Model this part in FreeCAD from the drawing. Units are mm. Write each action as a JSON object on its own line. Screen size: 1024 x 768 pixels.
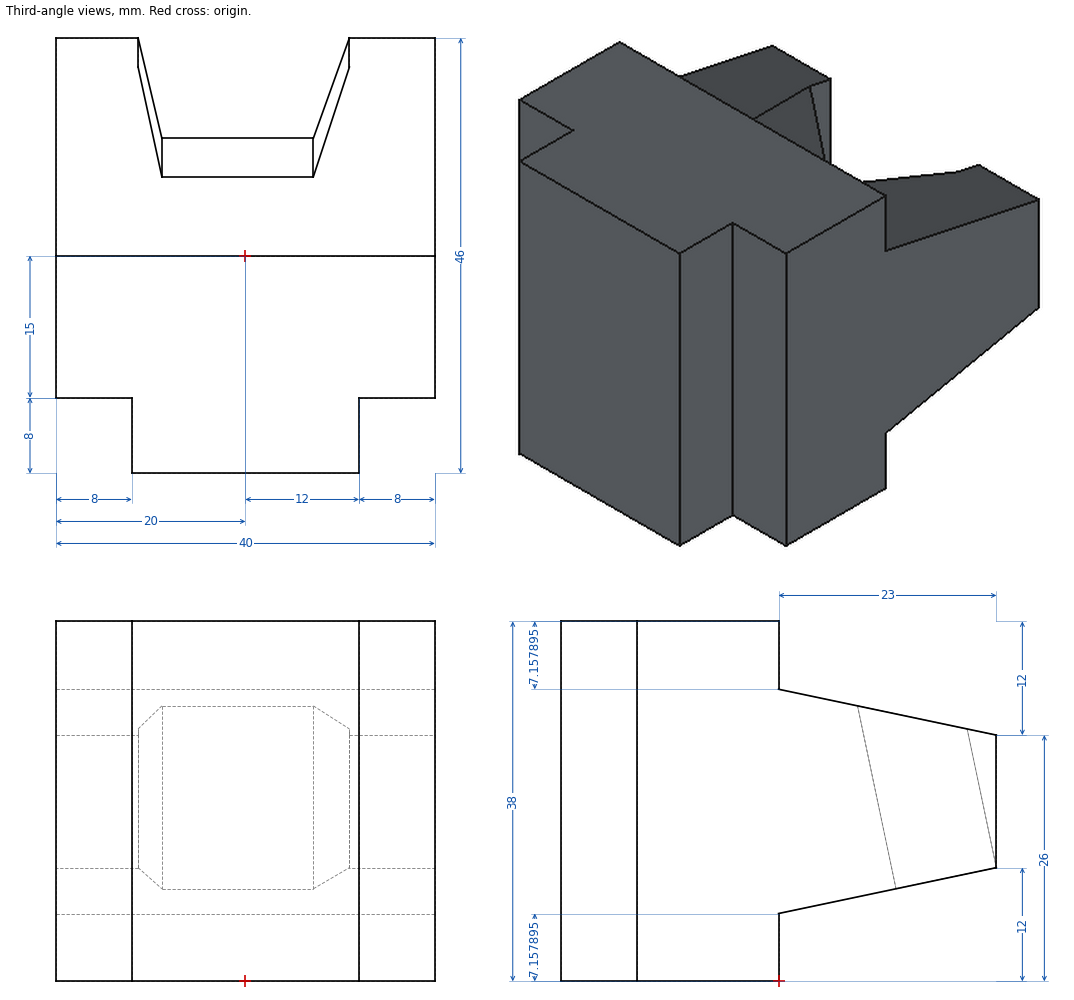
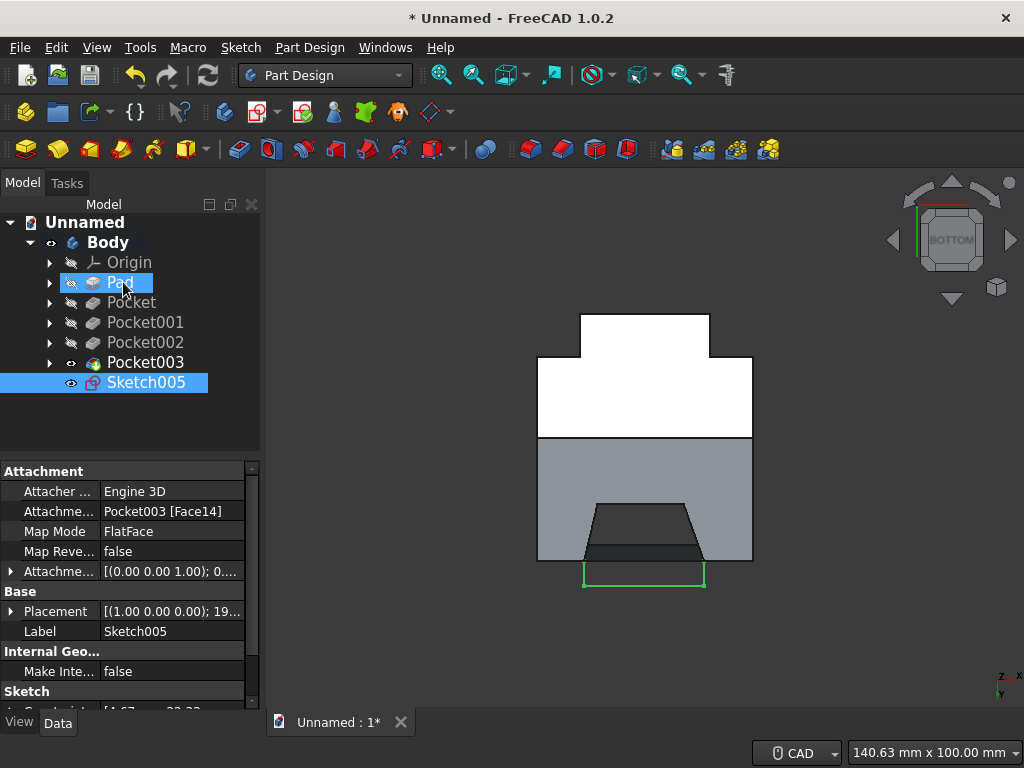
{"action": "left_click", "coordinate": [240, 150]}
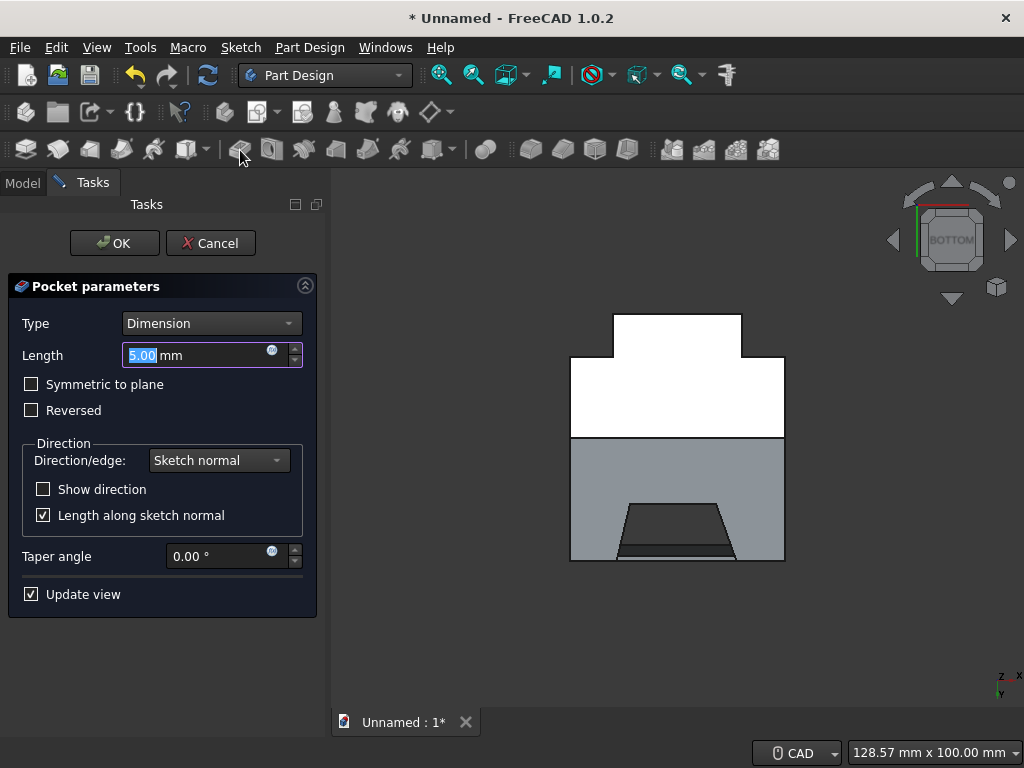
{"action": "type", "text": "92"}
{"action": "key", "text": "Tab"}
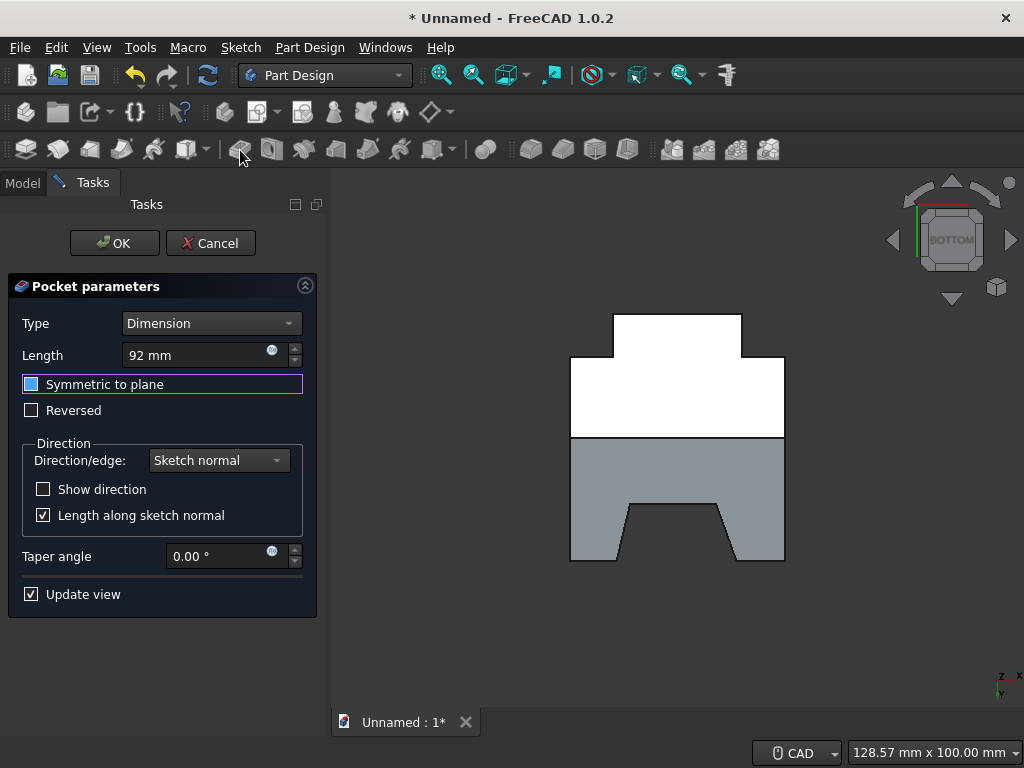
{"action": "left_click", "coordinate": [30, 384]}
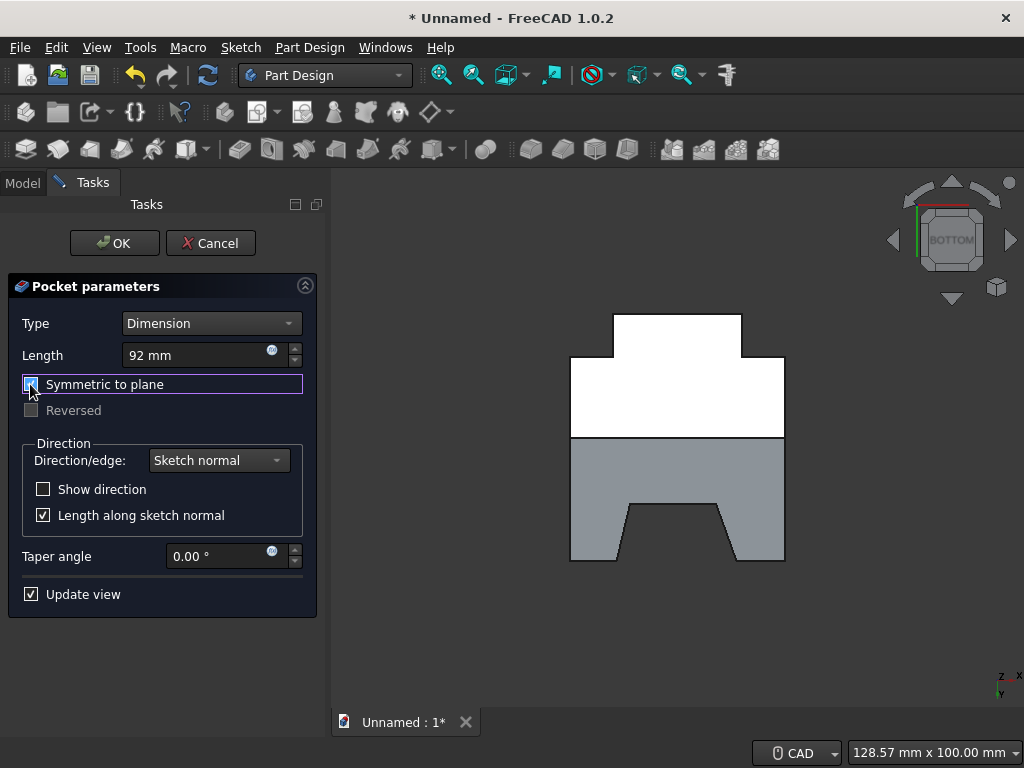
{"action": "left_click", "coordinate": [115, 243]}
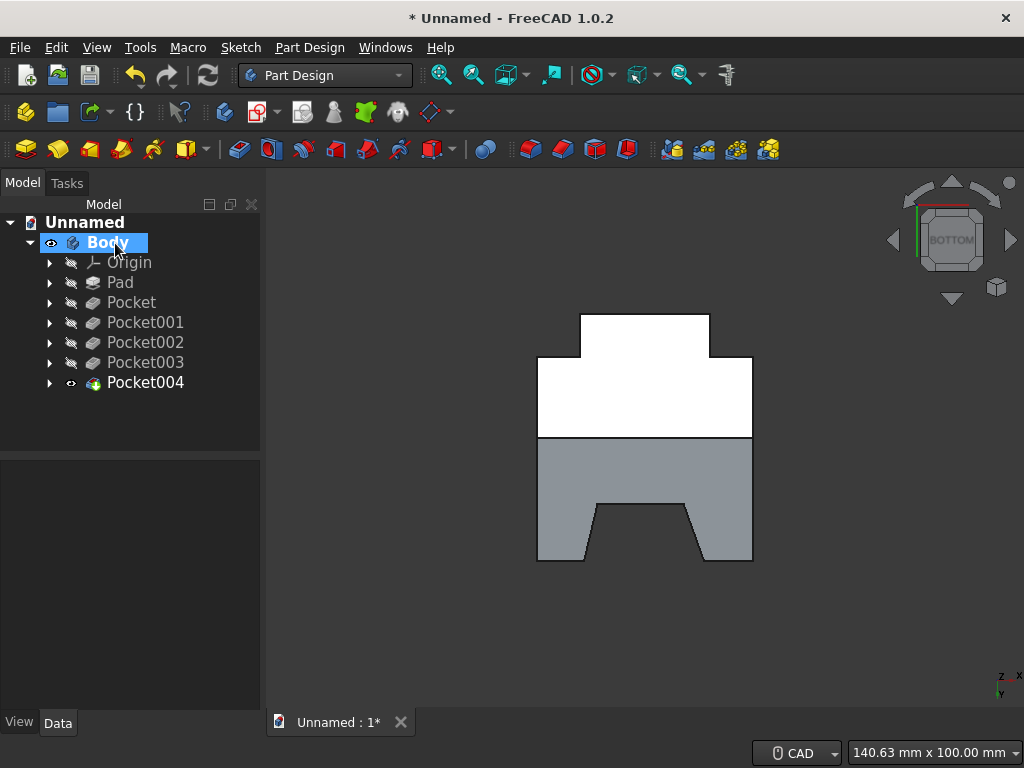
{"action": "key", "text": "0"}